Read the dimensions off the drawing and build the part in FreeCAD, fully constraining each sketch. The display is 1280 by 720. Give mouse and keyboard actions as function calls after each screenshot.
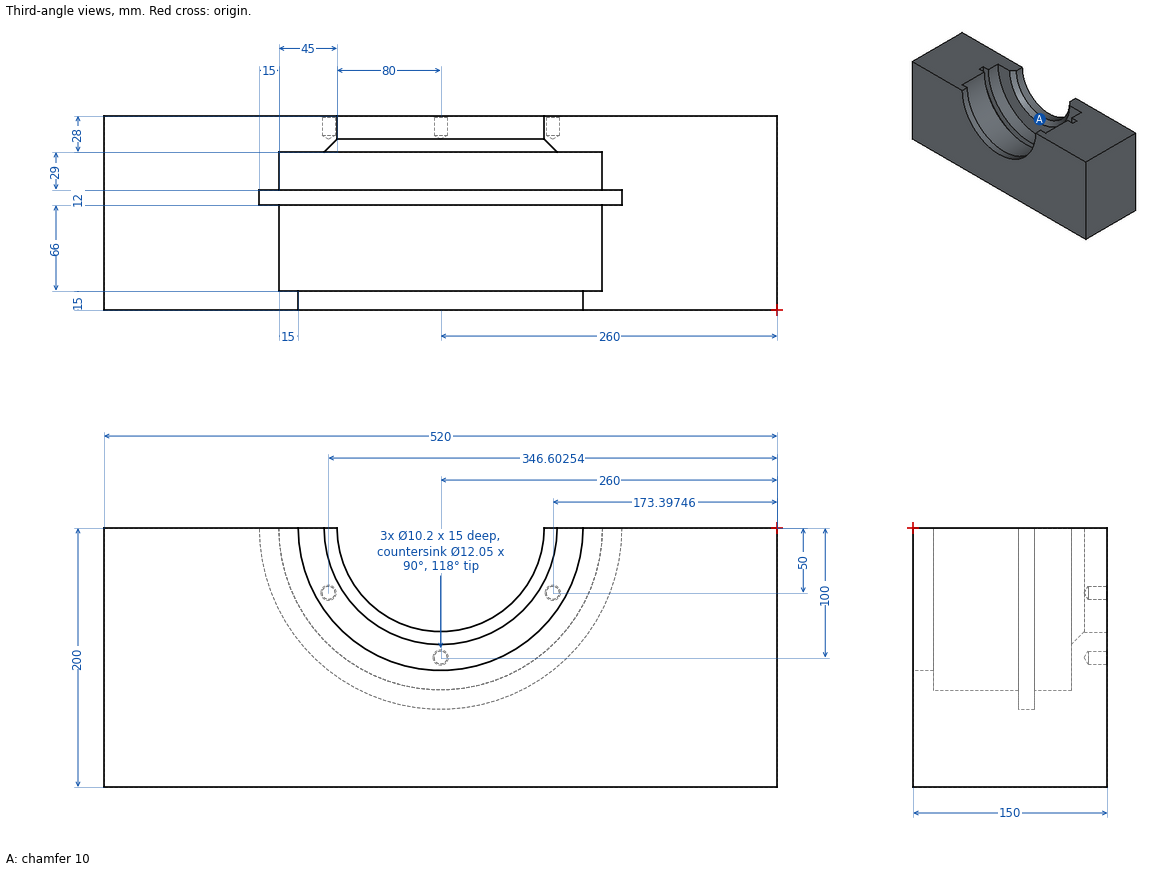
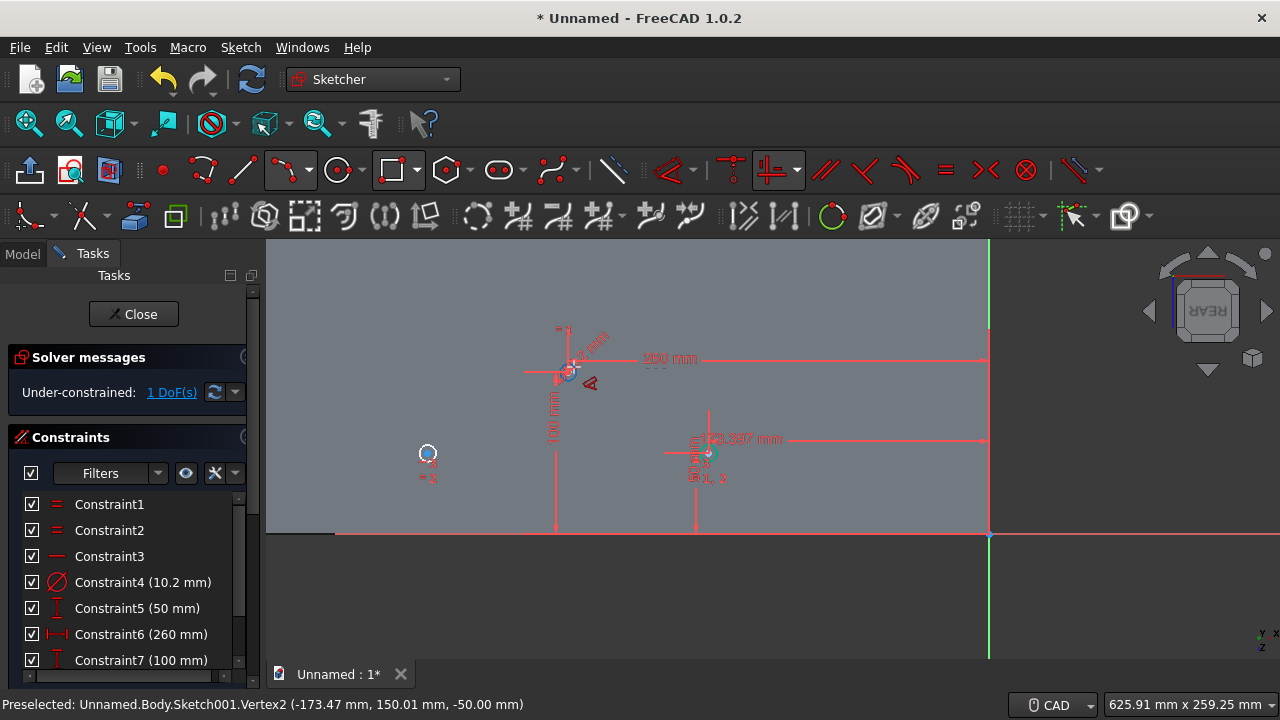
click(428, 453)
click(709, 568)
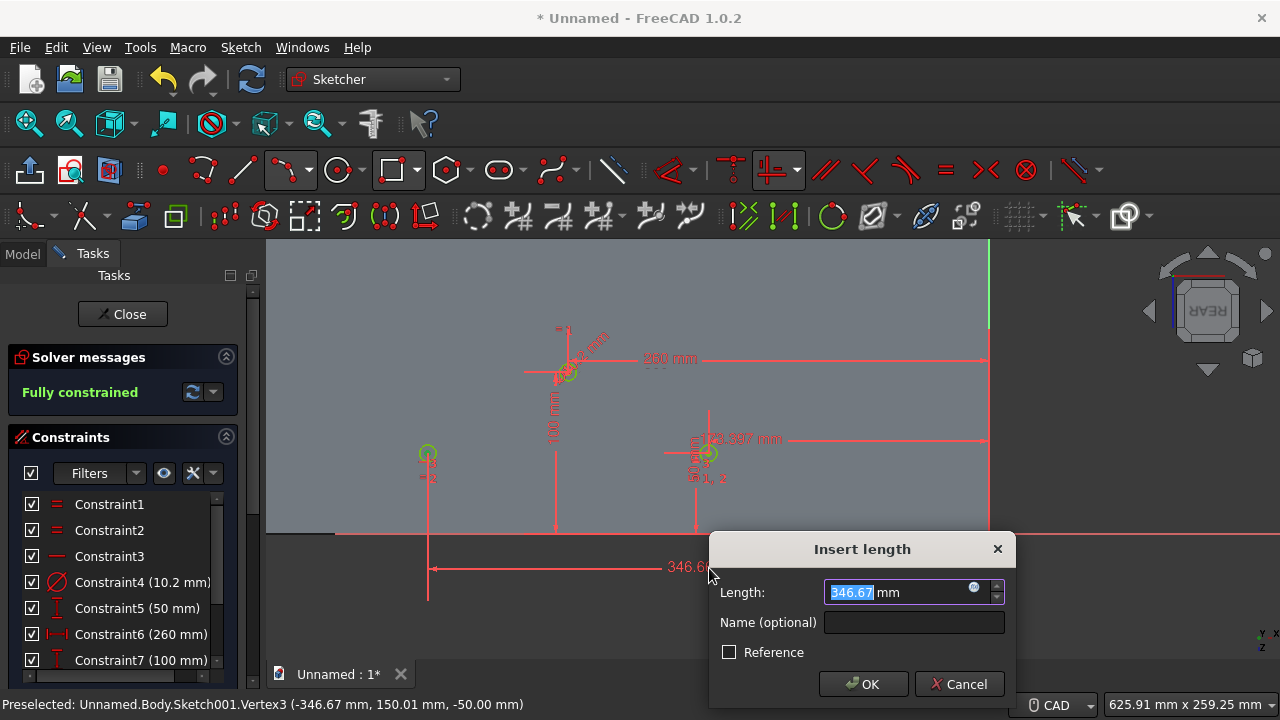
text(346.60254)
key(Return)
key(Escape)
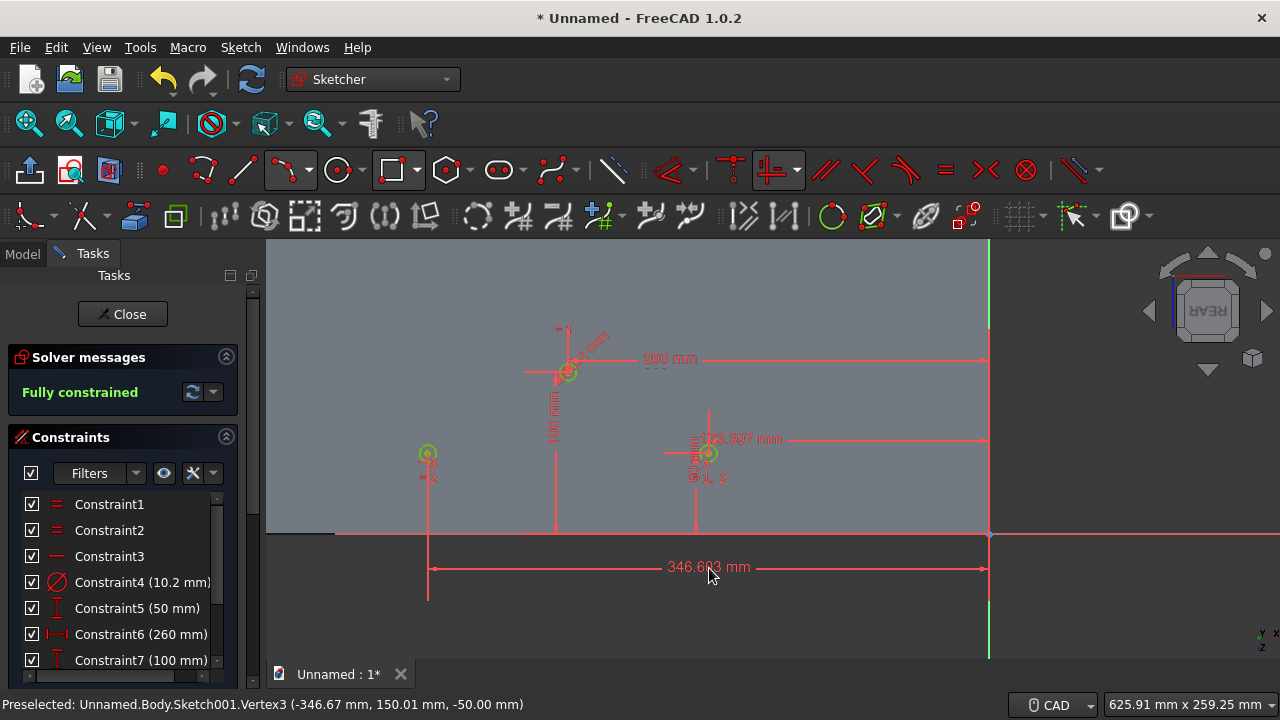
click(123, 314)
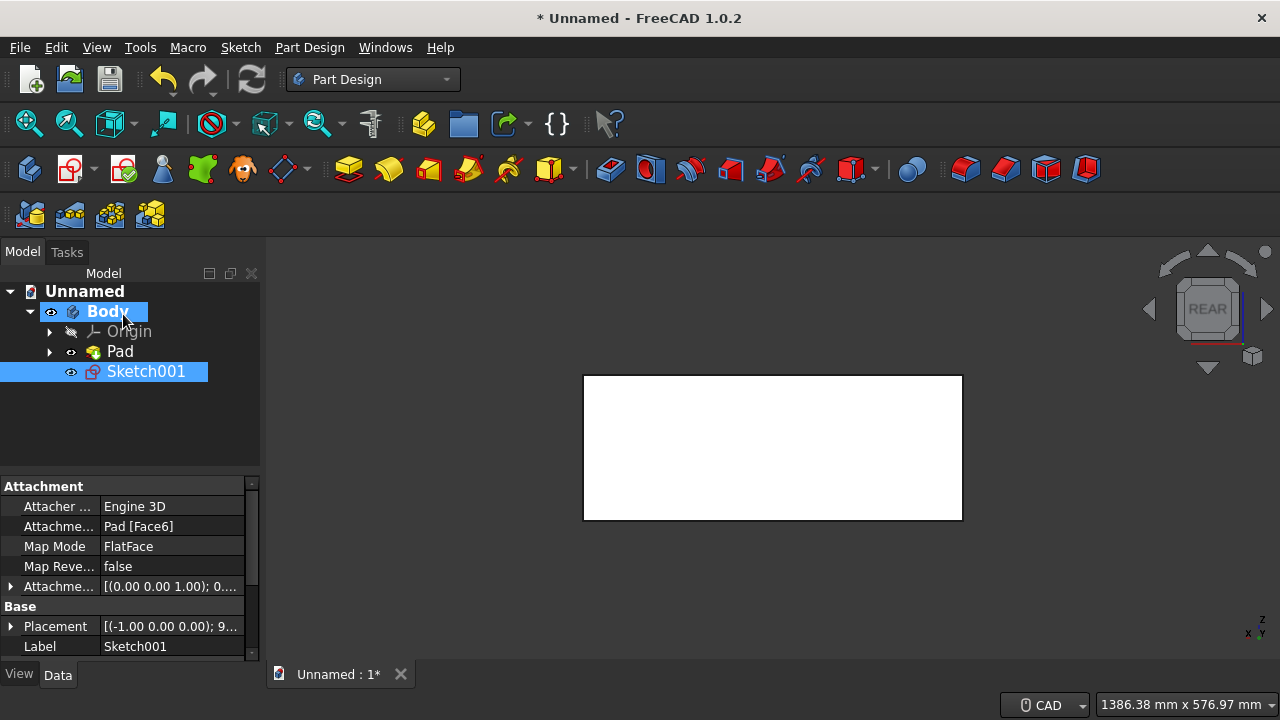
click(652, 170)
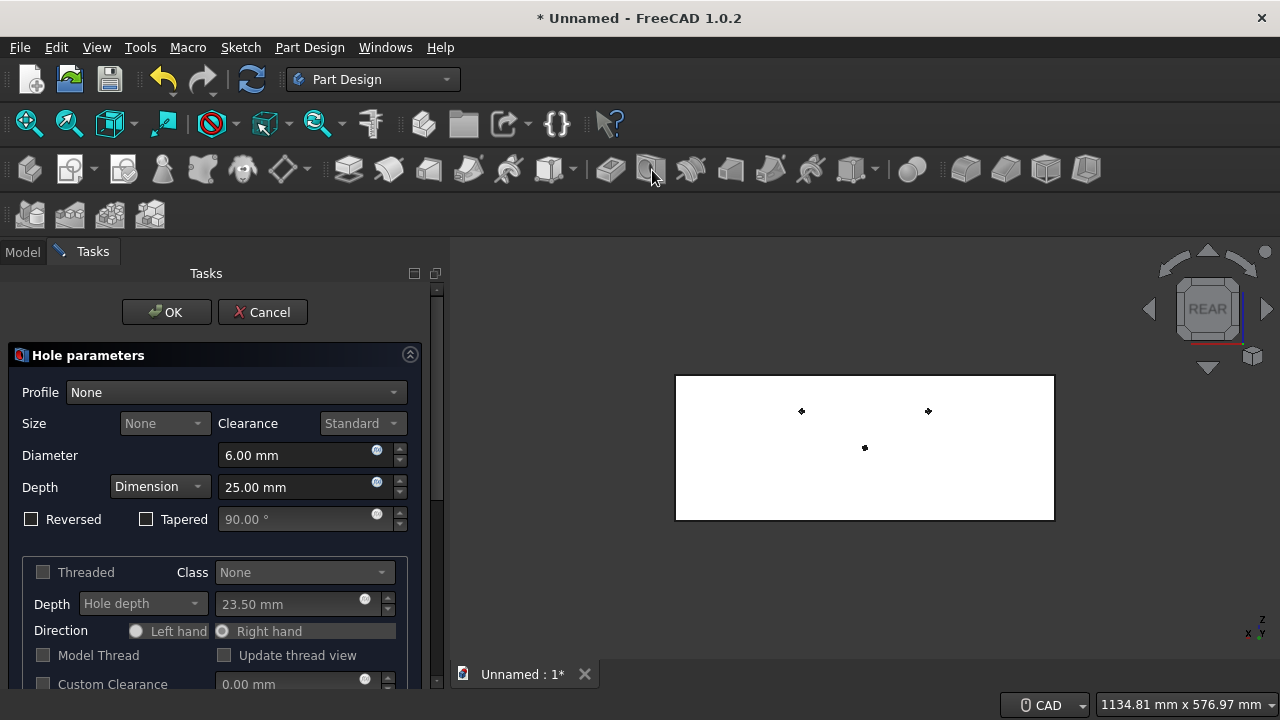
triple_click(305, 455)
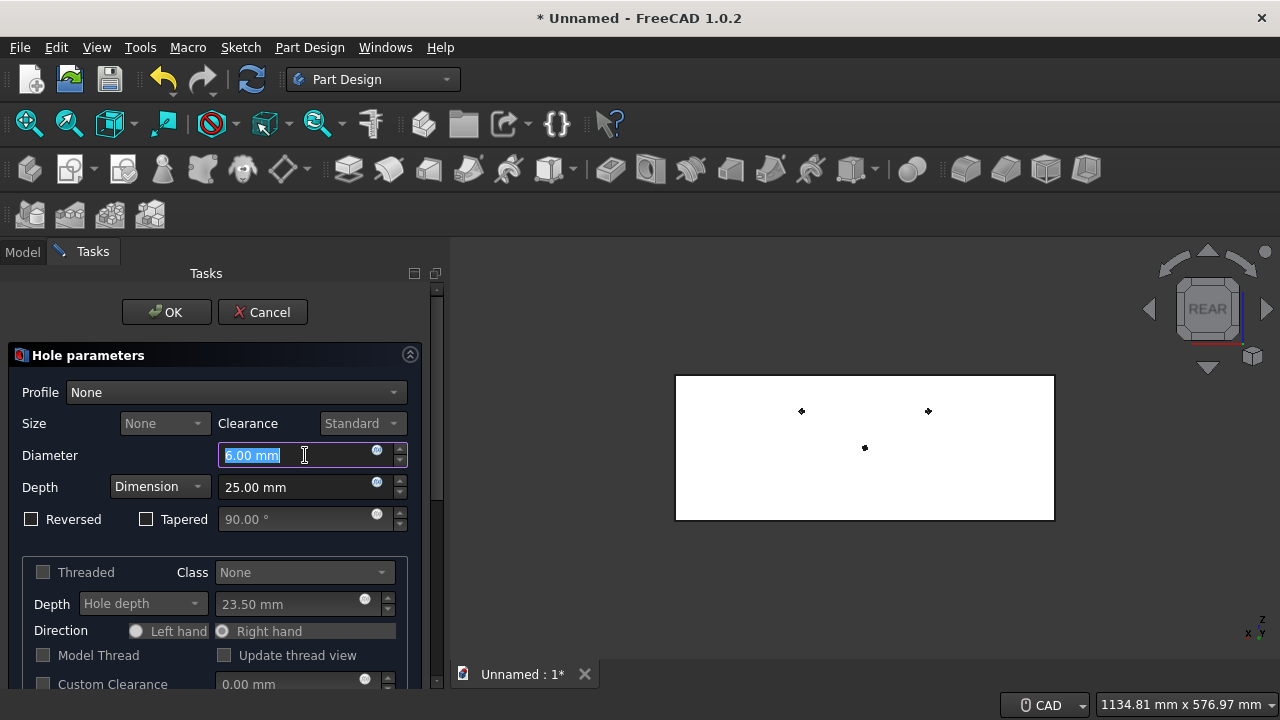
text(10.2)
key(Tab)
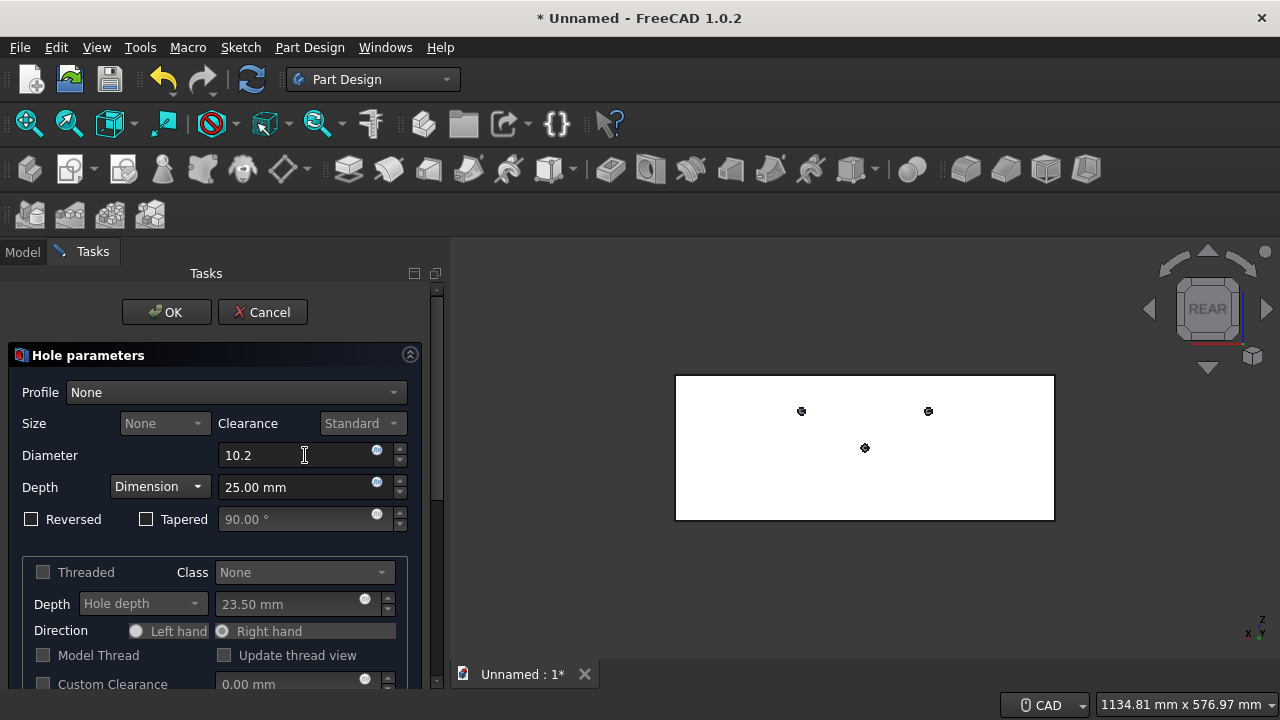
triple_click(305, 487)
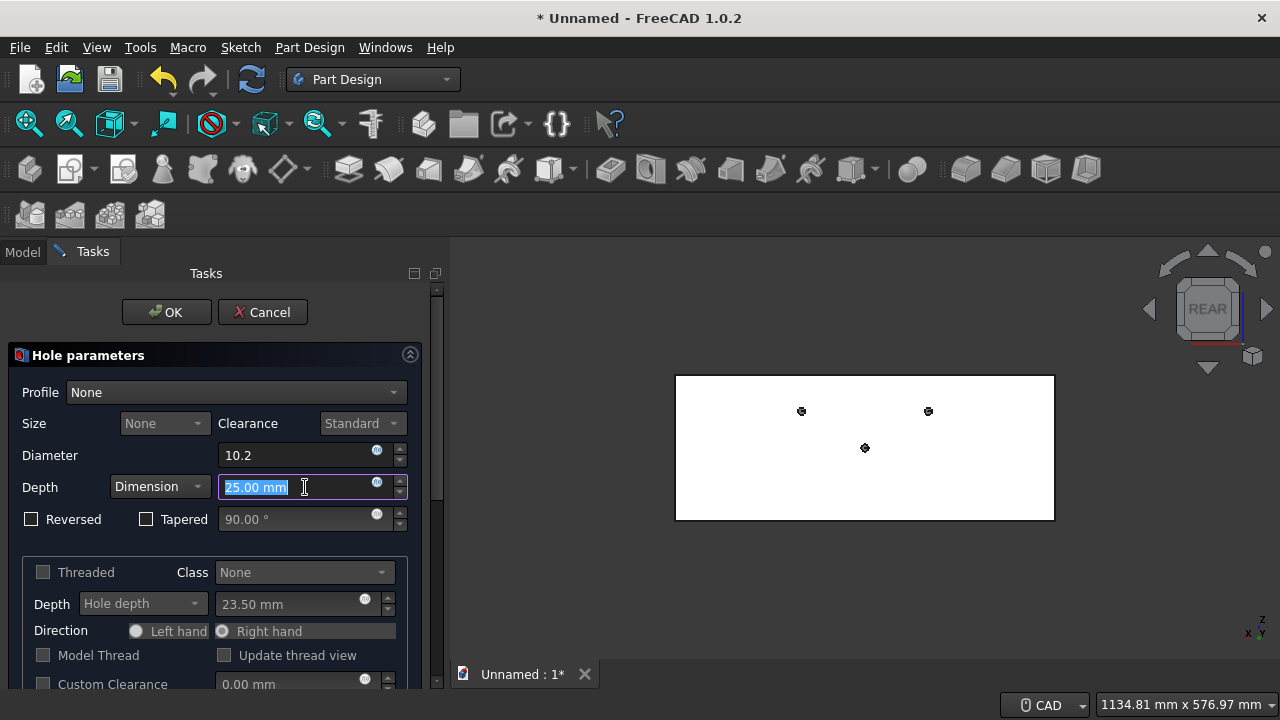
text(15)
key(Tab)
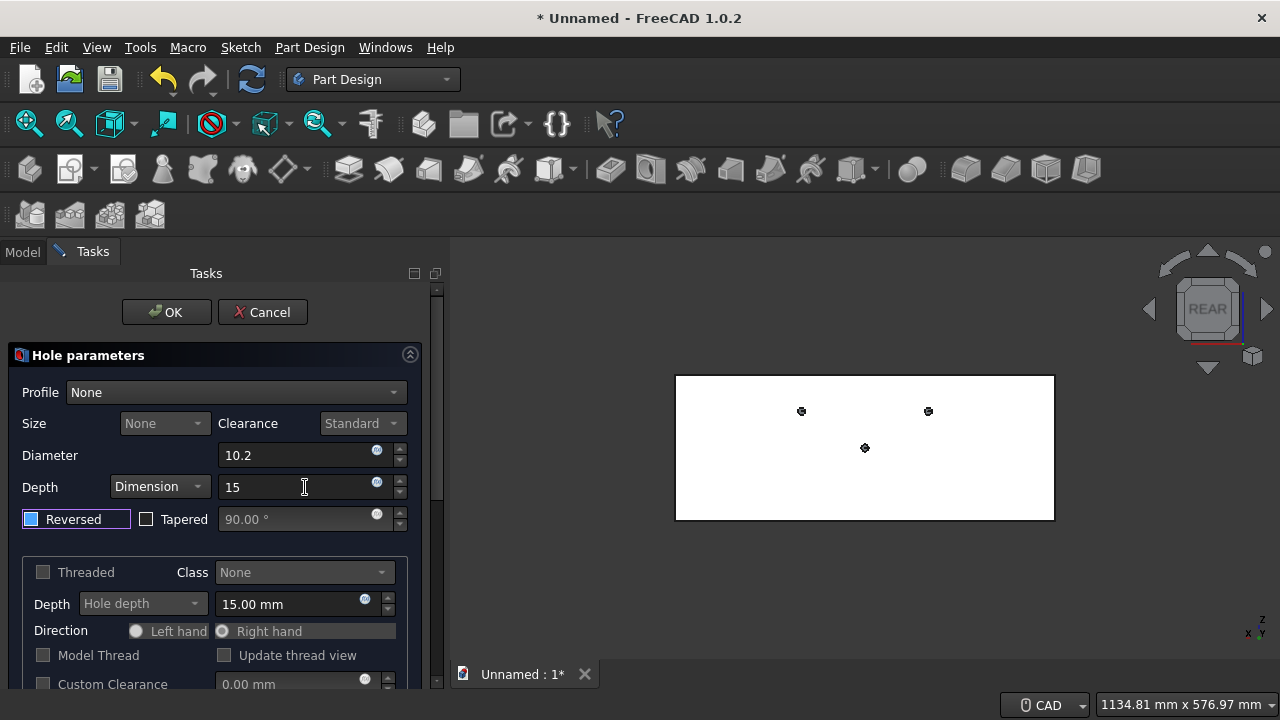
scroll(437, 486, down, 3)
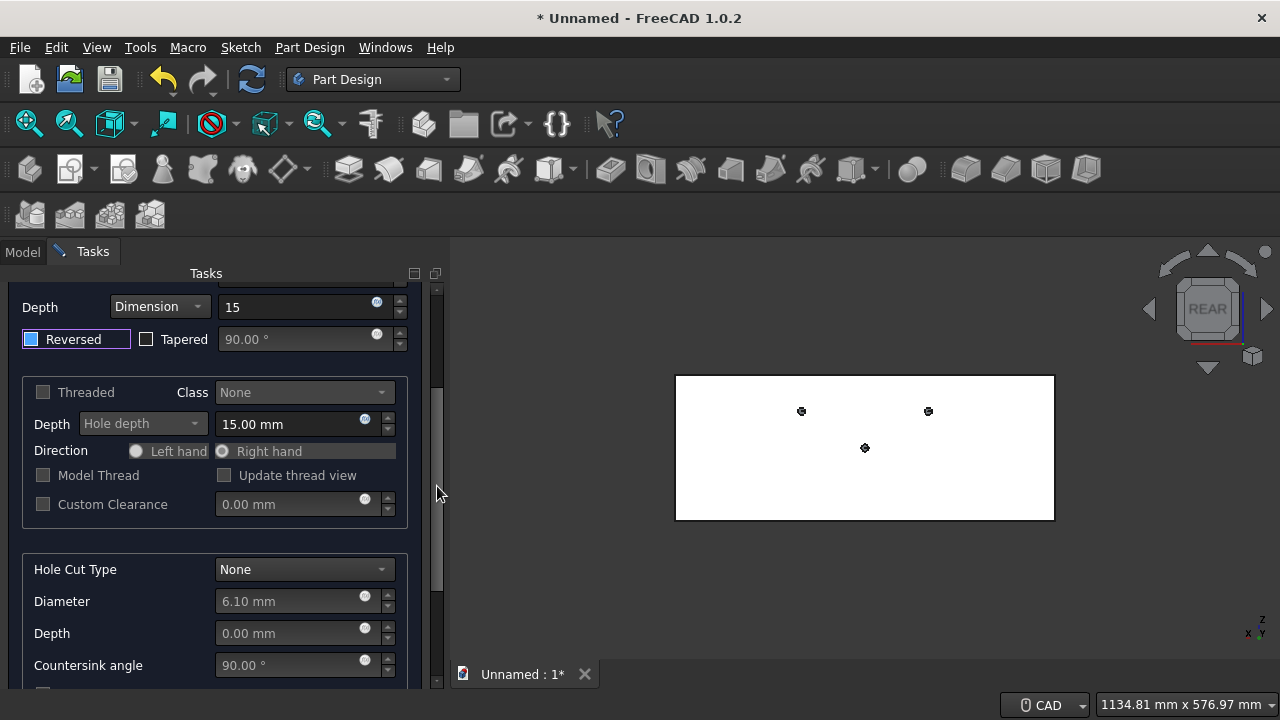
click(306, 570)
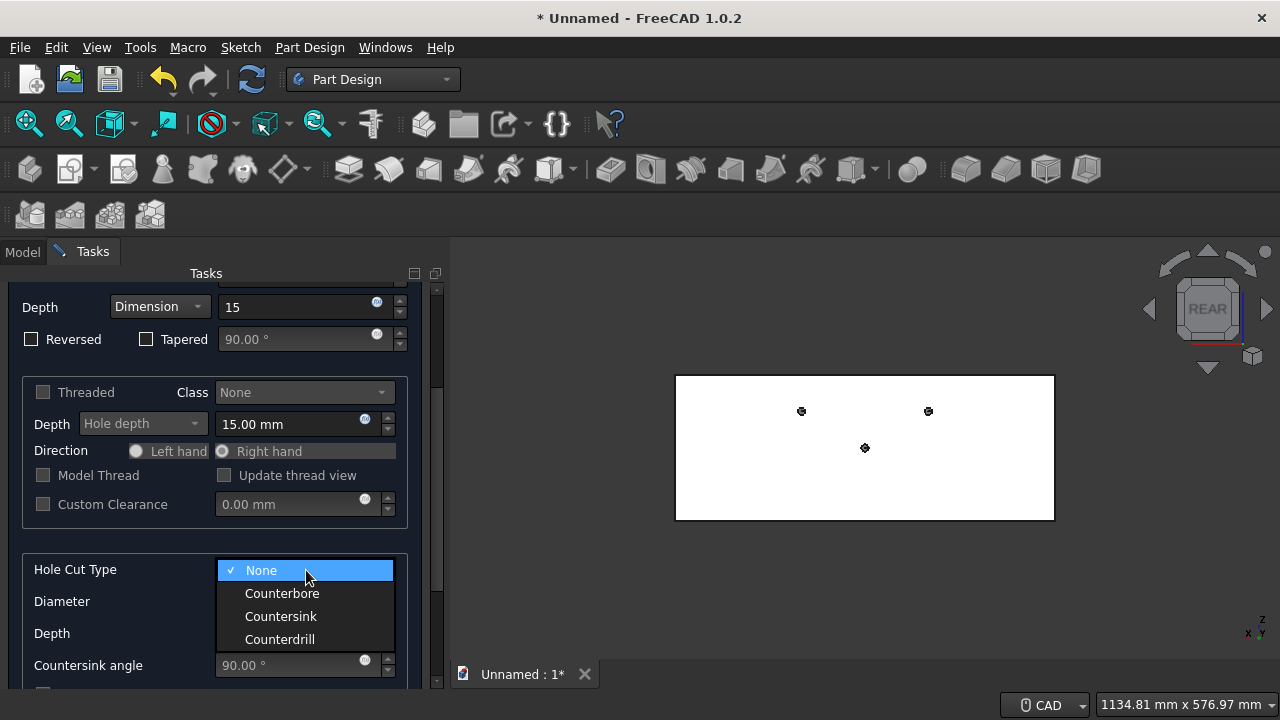
click(304, 616)